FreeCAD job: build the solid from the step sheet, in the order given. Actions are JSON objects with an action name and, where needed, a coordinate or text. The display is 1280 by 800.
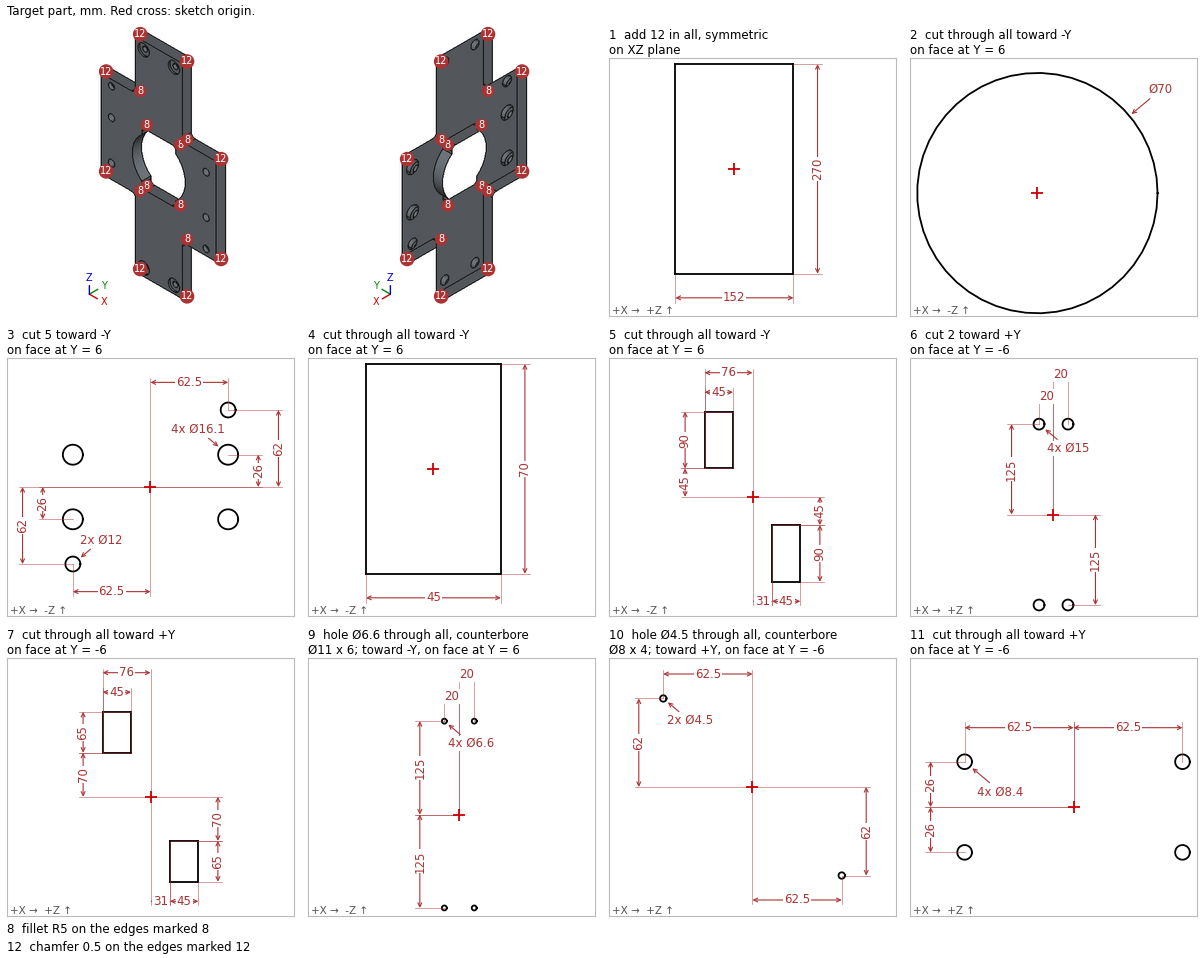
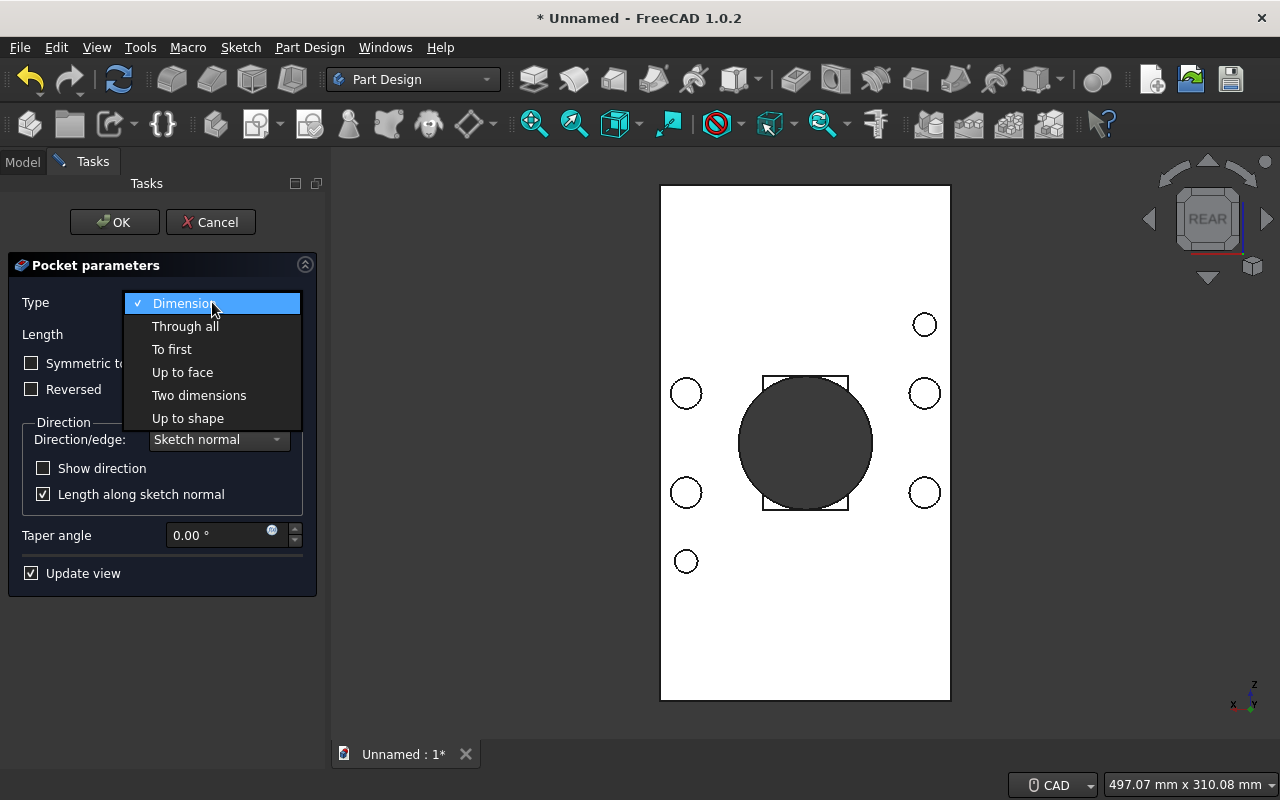
{"action": "left_click", "coordinate": [212, 326]}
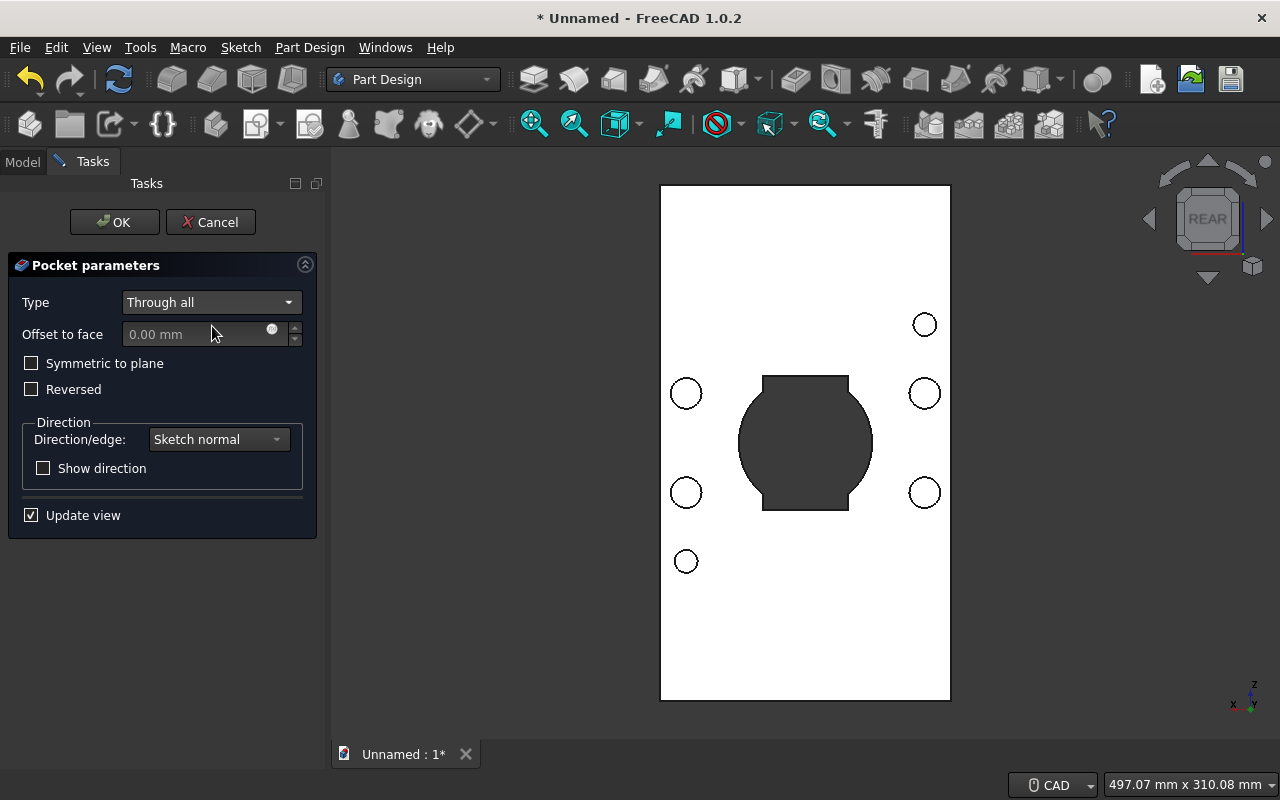
{"action": "left_click", "coordinate": [115, 222]}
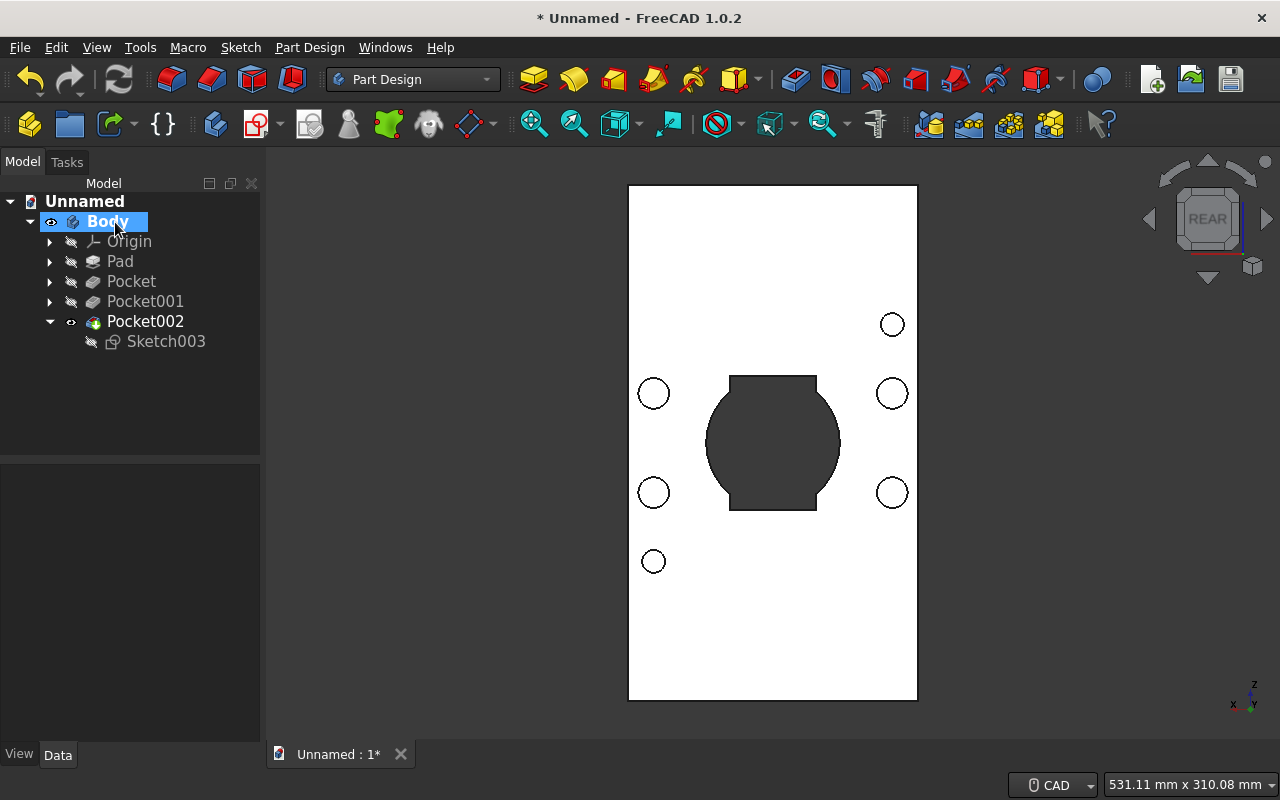
{"action": "left_click", "coordinate": [732, 295]}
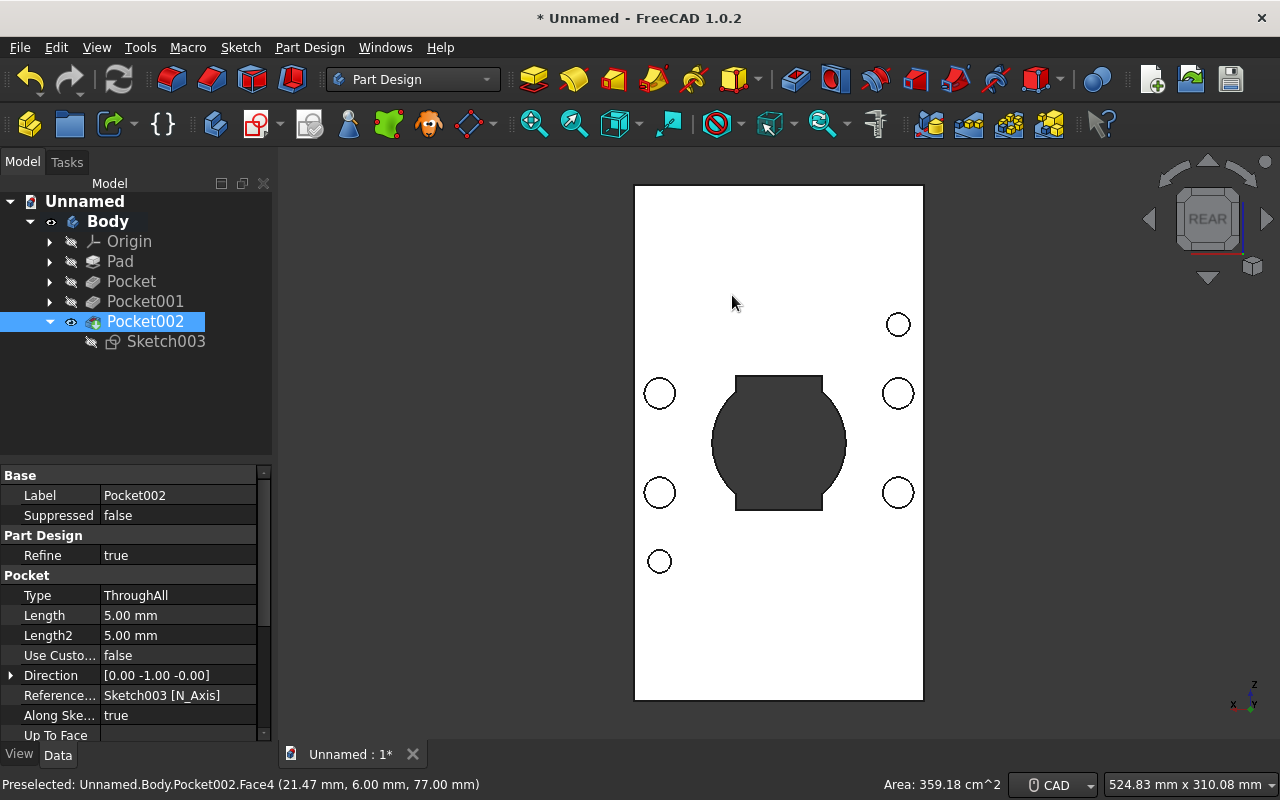
{"action": "left_click", "coordinate": [256, 124]}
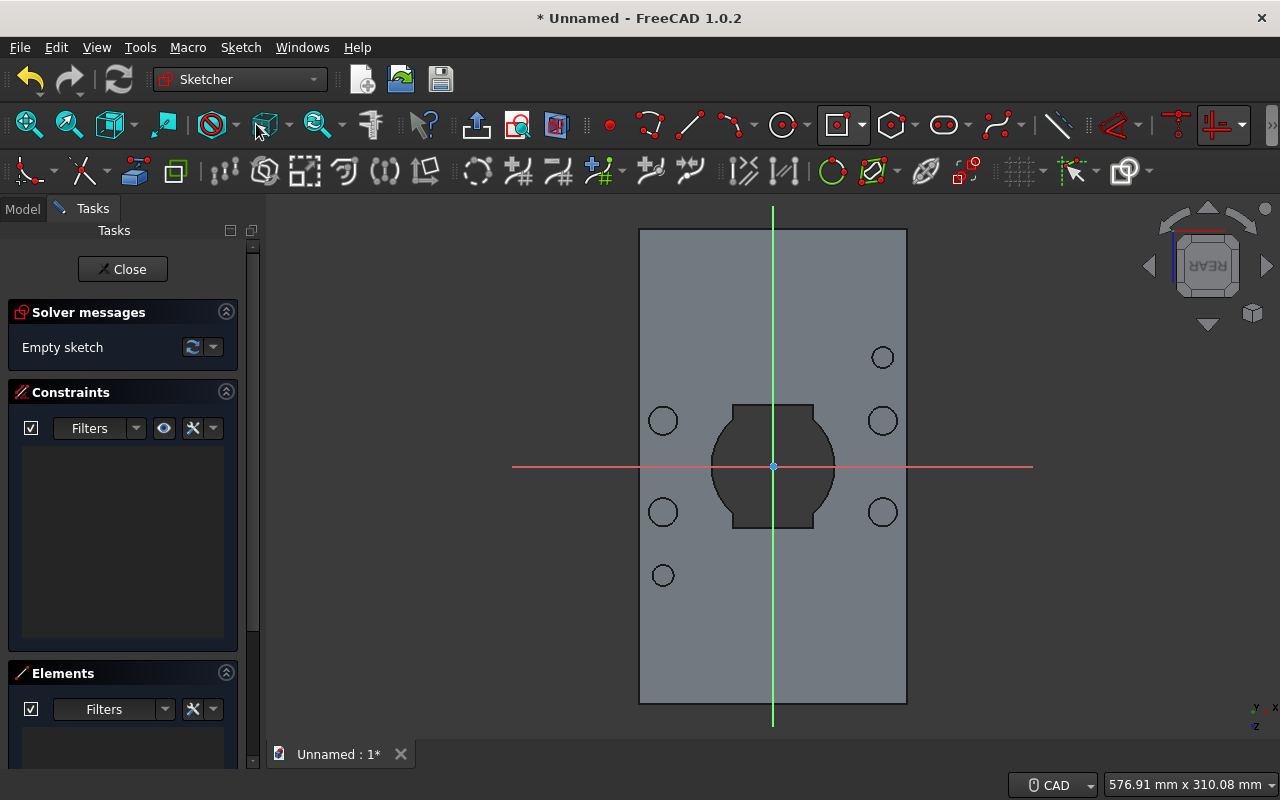
{"action": "scroll", "coordinate": [565, 467], "scroll_direction": "down", "scroll_amount": 2}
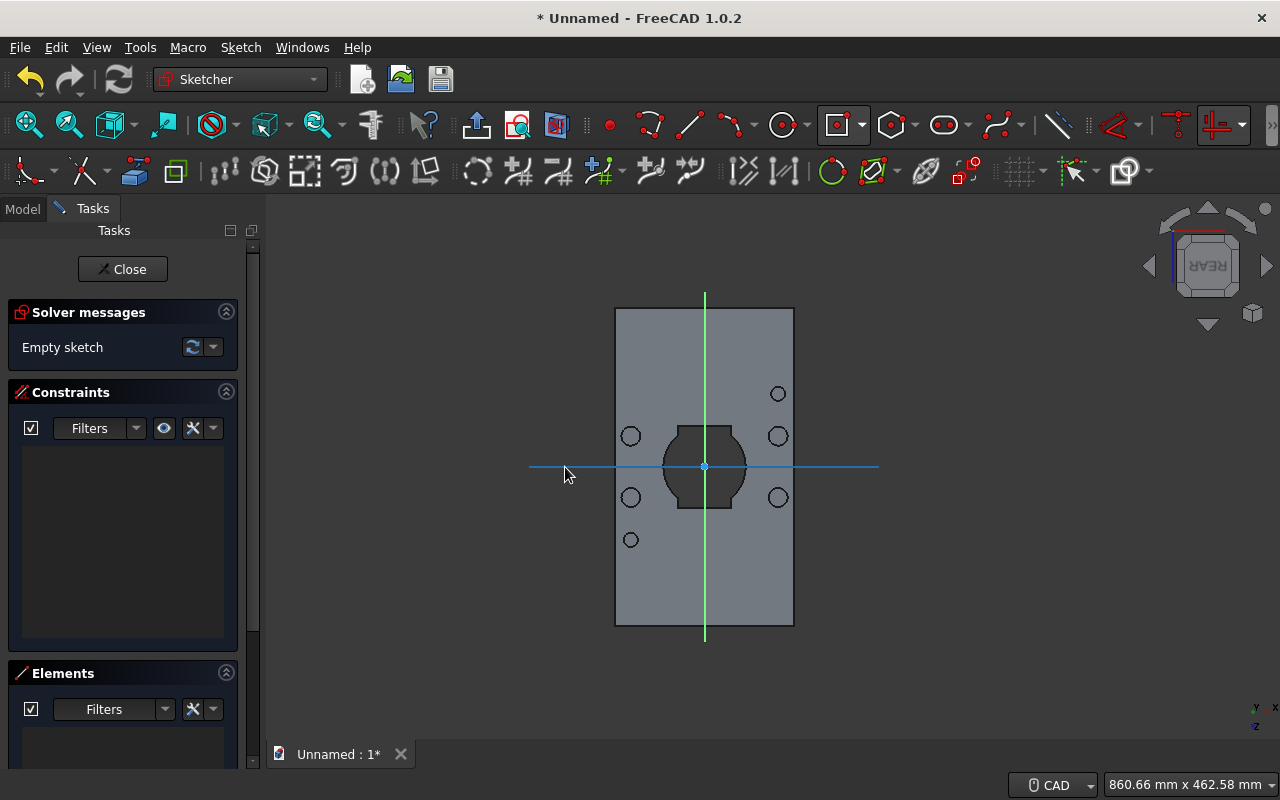
{"action": "key", "text": "g r"}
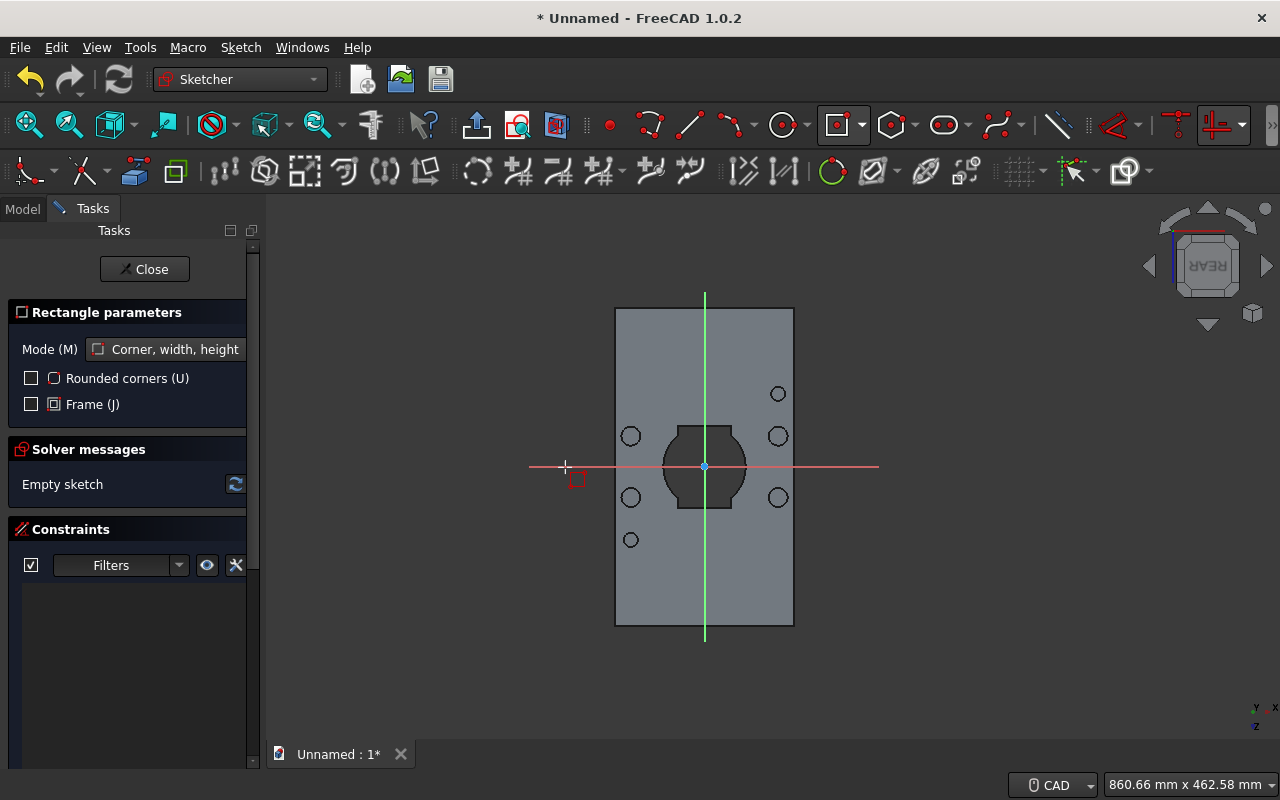
{"action": "left_click", "coordinate": [615, 308]}
{"action": "mouse_move", "coordinate": [668, 414]}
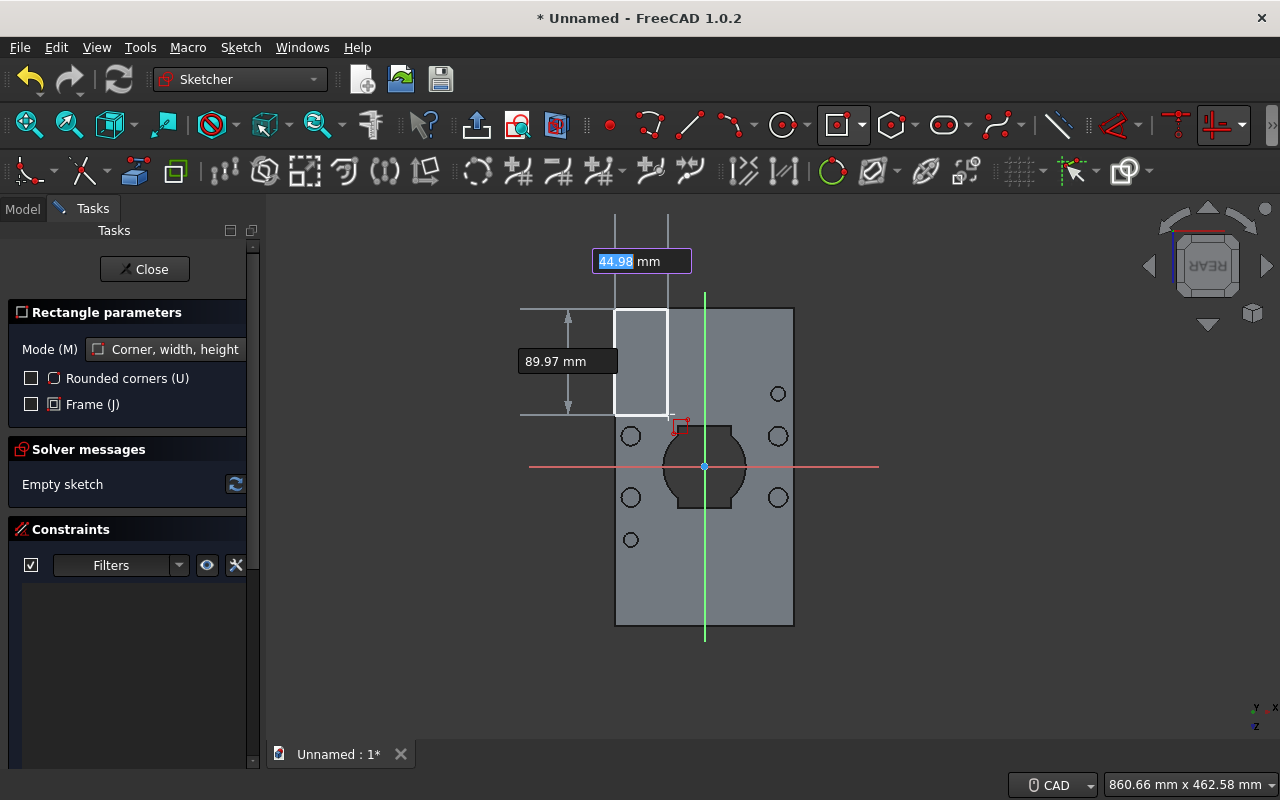
{"action": "type", "text": "45"}
{"action": "key", "text": "Tab"}
{"action": "type", "text": "90"}
{"action": "key", "text": "Return"}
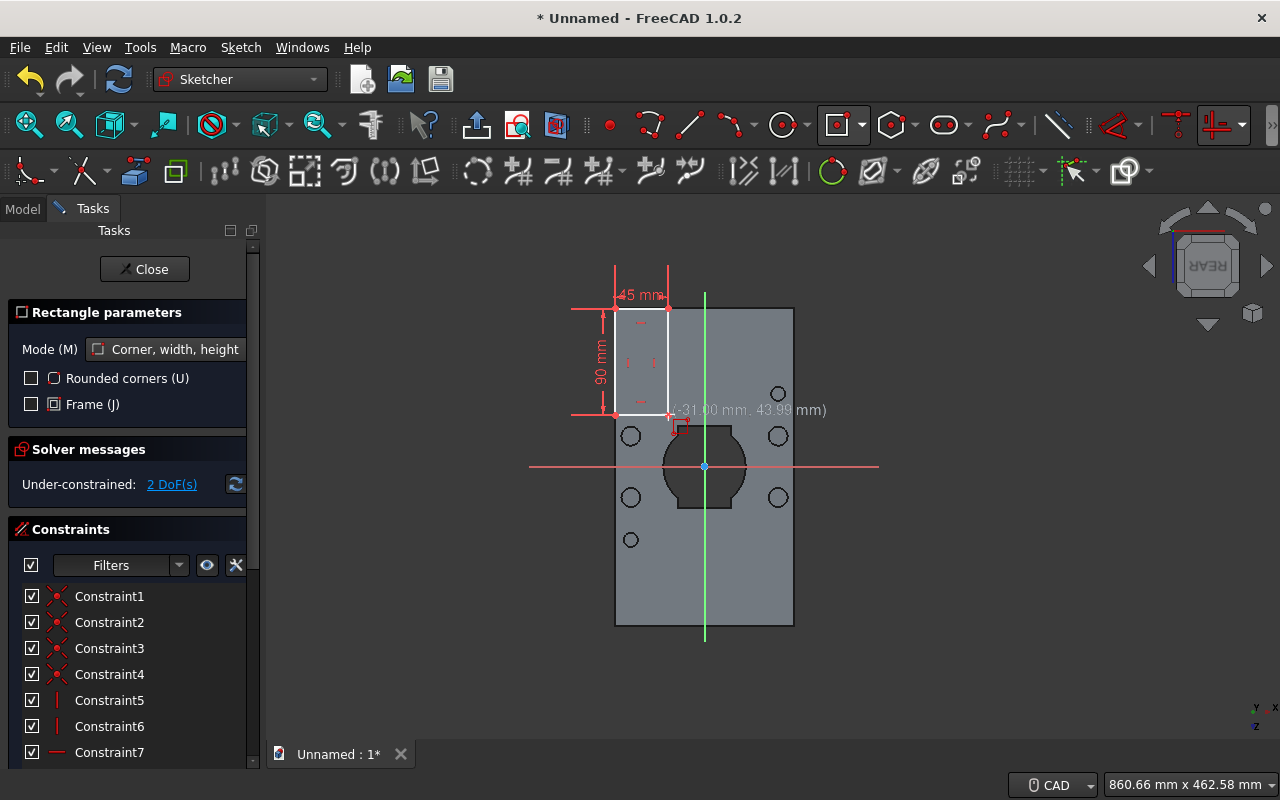
{"action": "left_click", "coordinate": [741, 520]}
{"action": "mouse_move", "coordinate": [794, 626]}